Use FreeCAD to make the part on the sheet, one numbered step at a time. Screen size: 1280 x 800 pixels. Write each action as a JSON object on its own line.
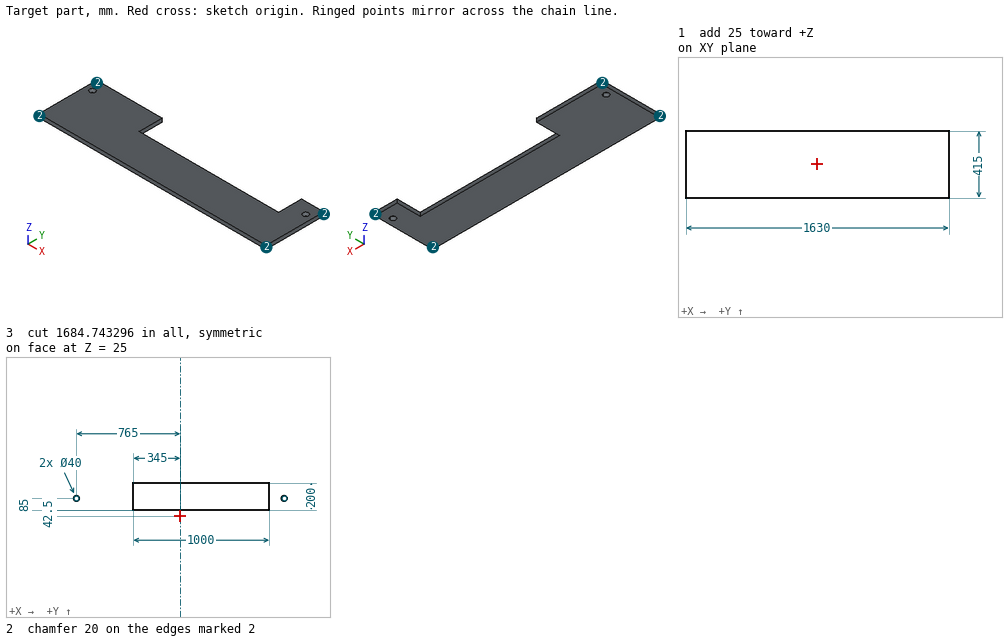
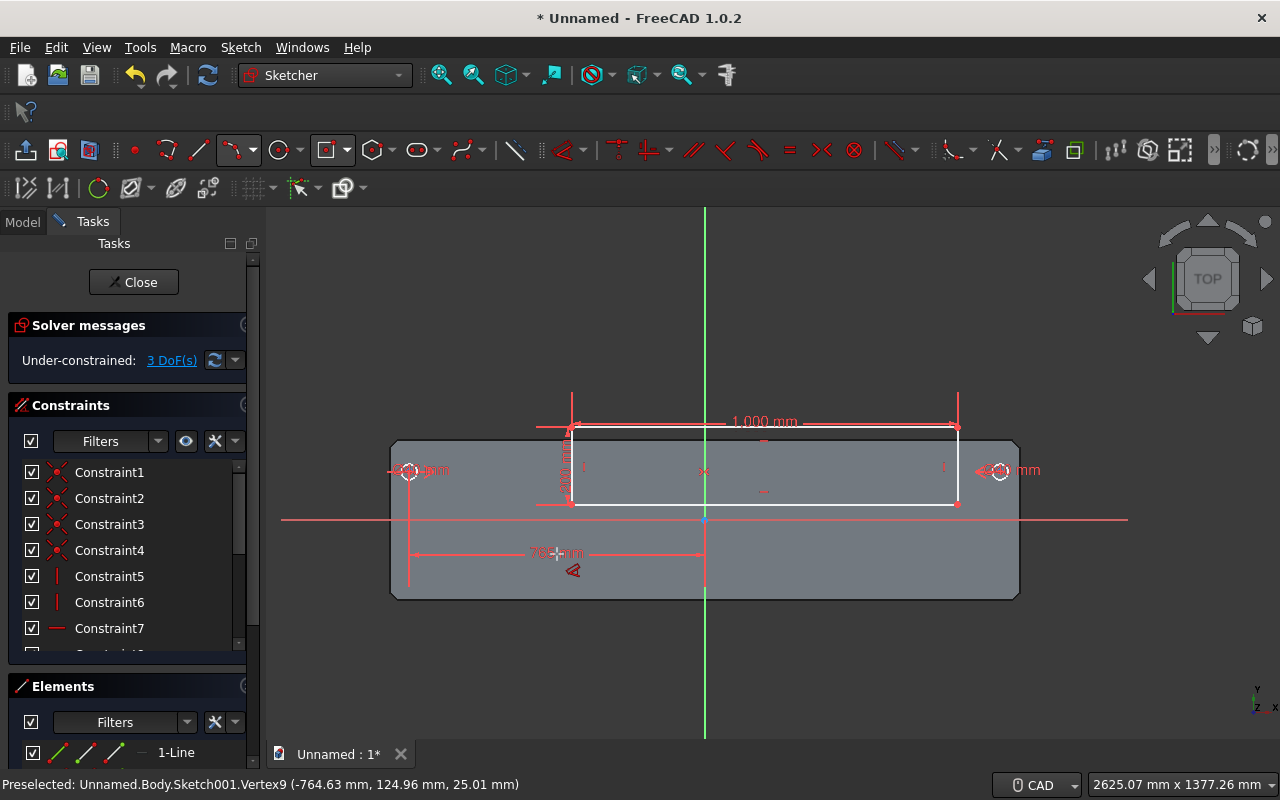
{"action": "left_click", "coordinate": [572, 505]}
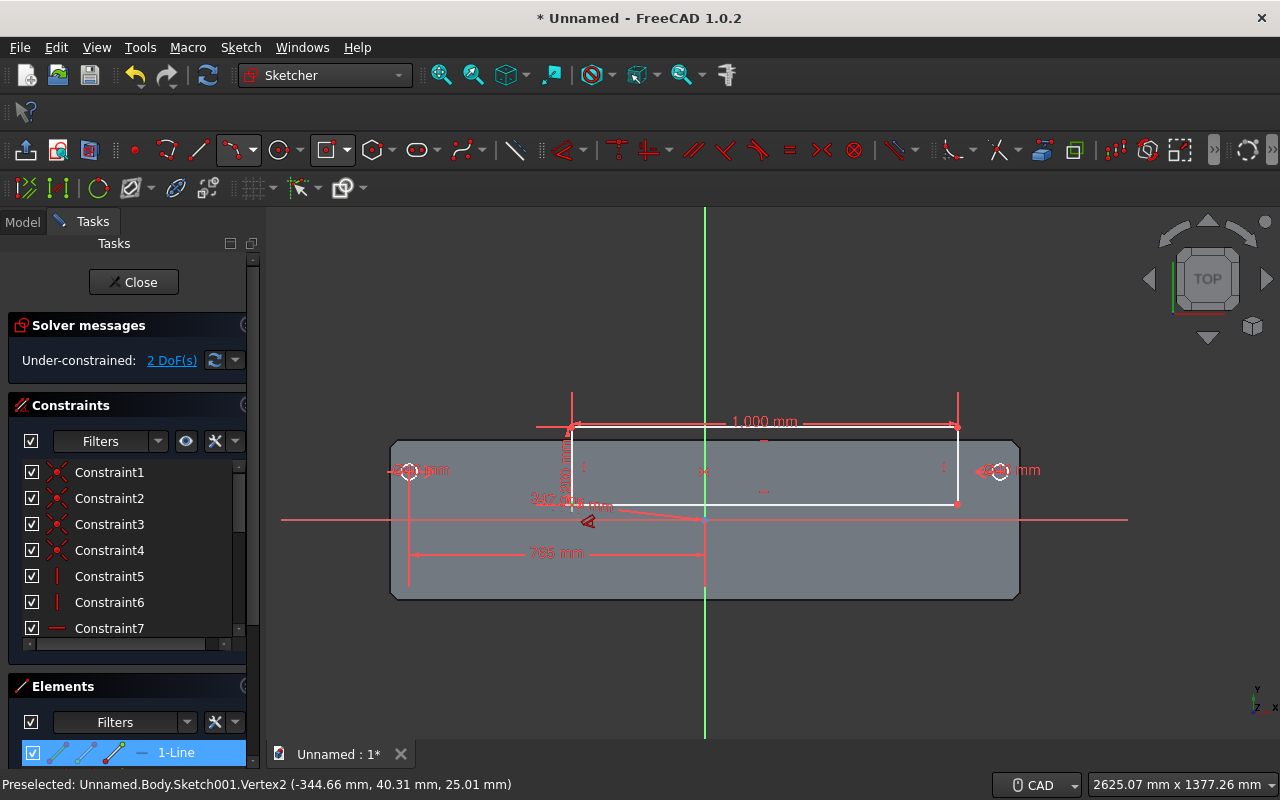
{"action": "left_click", "coordinate": [409, 472]}
{"action": "left_click", "coordinate": [375, 488]}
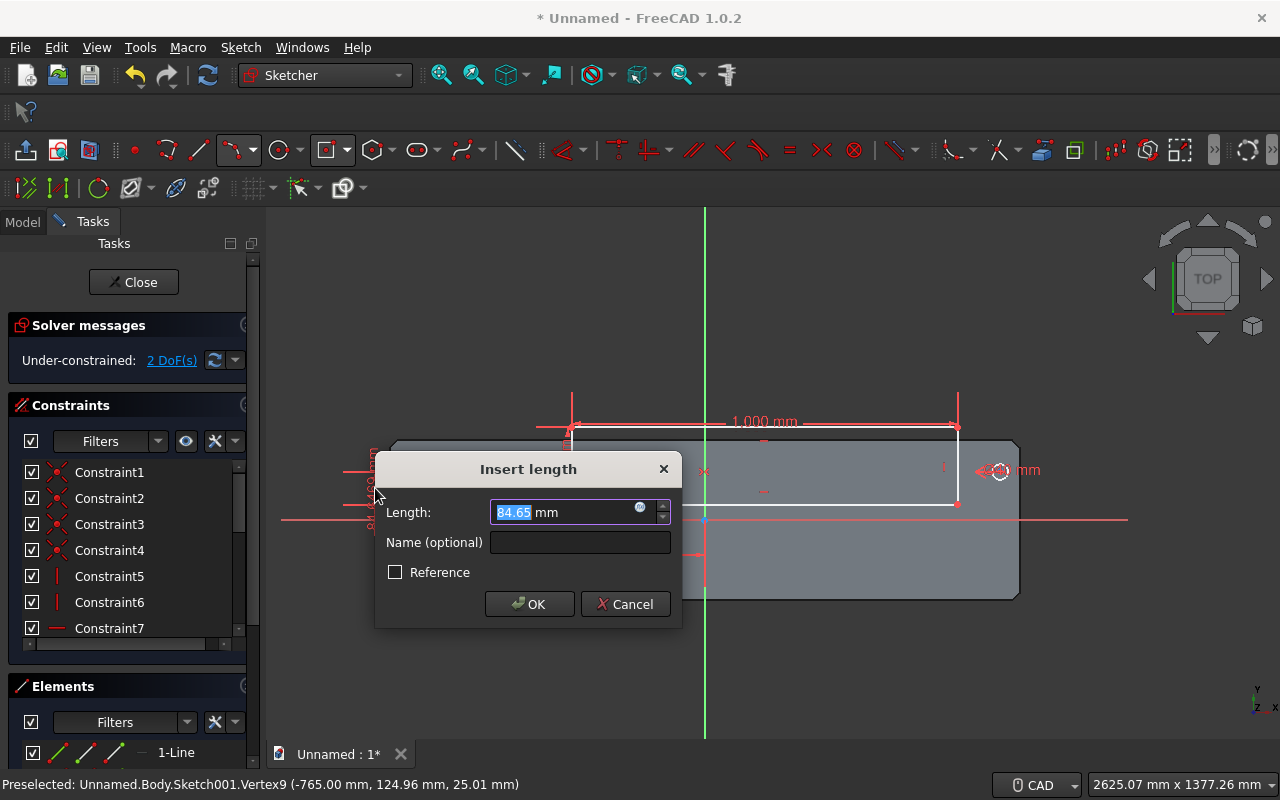
{"action": "type", "text": "85"}
{"action": "key", "text": "Return"}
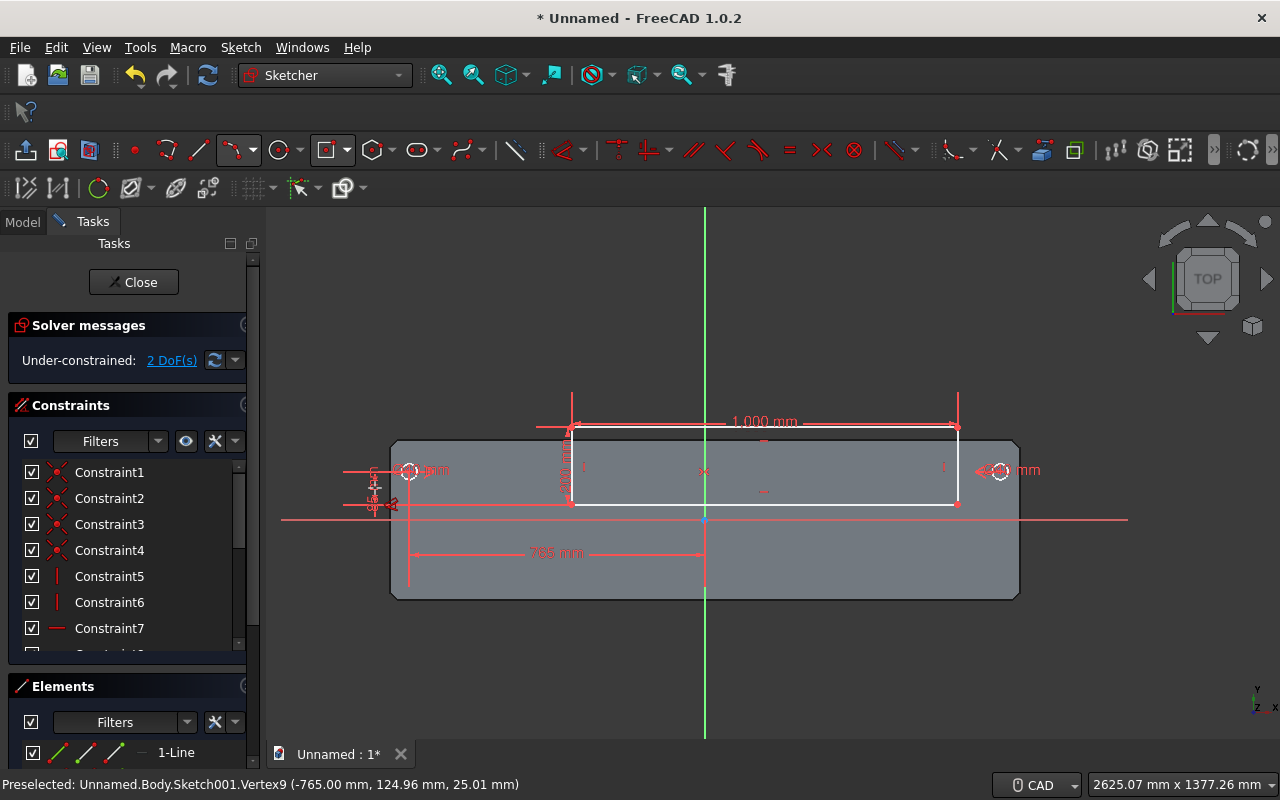
{"action": "left_click", "coordinate": [572, 427]}
{"action": "left_click", "coordinate": [638, 554]}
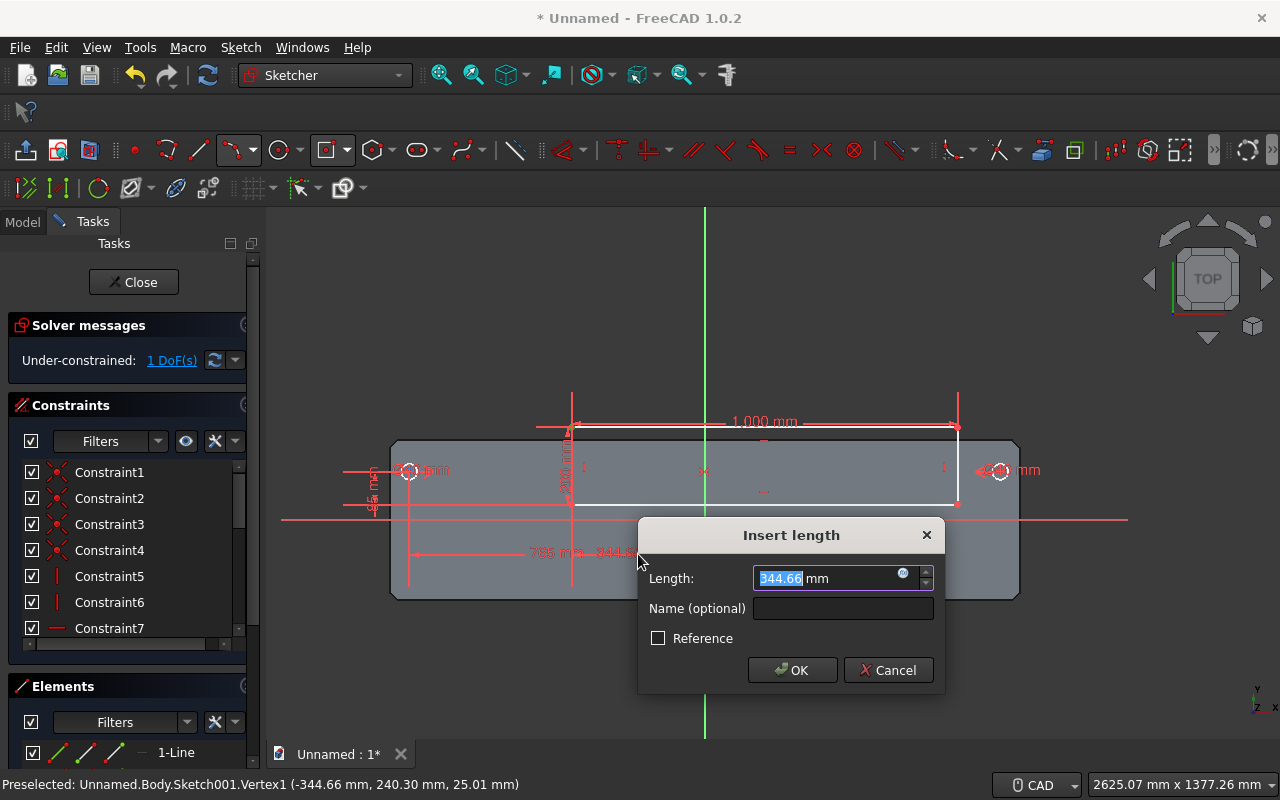
{"action": "type", "text": "345"}
{"action": "key", "text": "Return"}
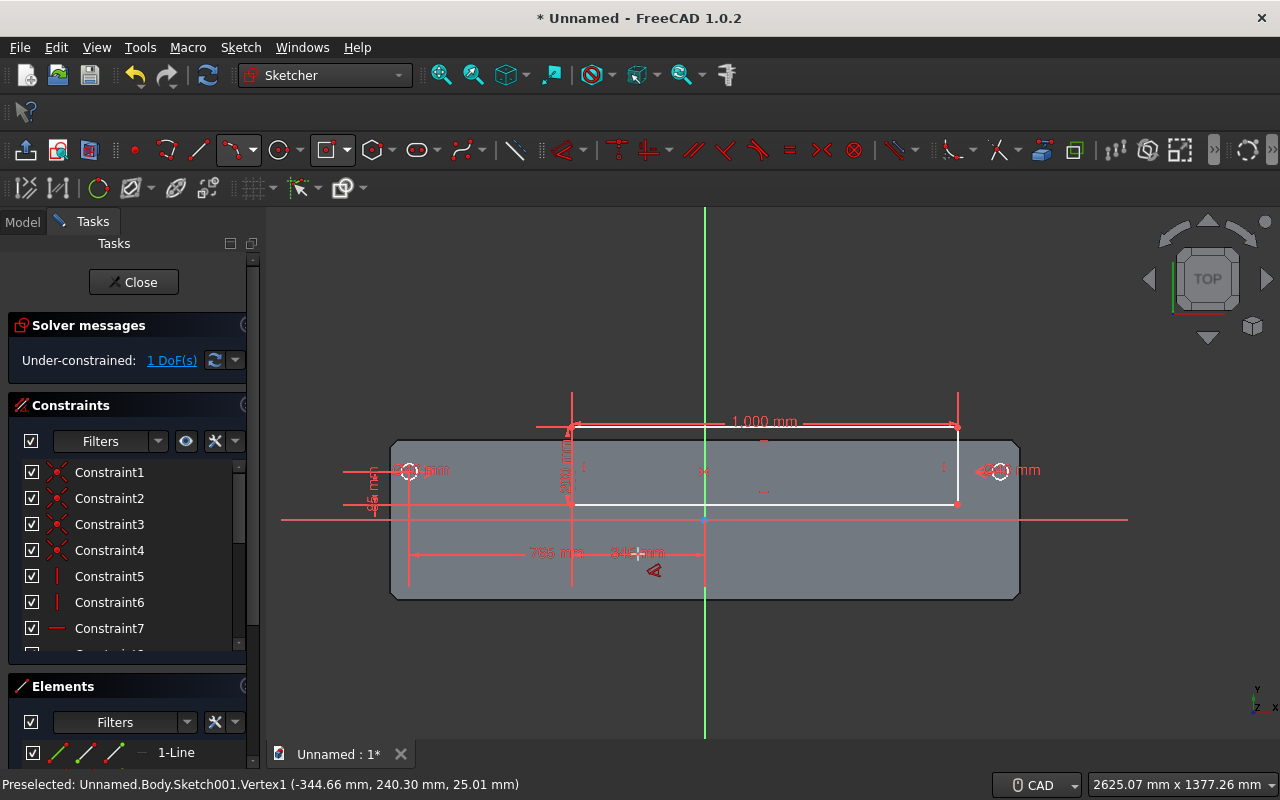
{"action": "scroll", "coordinate": [572, 505], "scroll_direction": "up", "scroll_amount": 5}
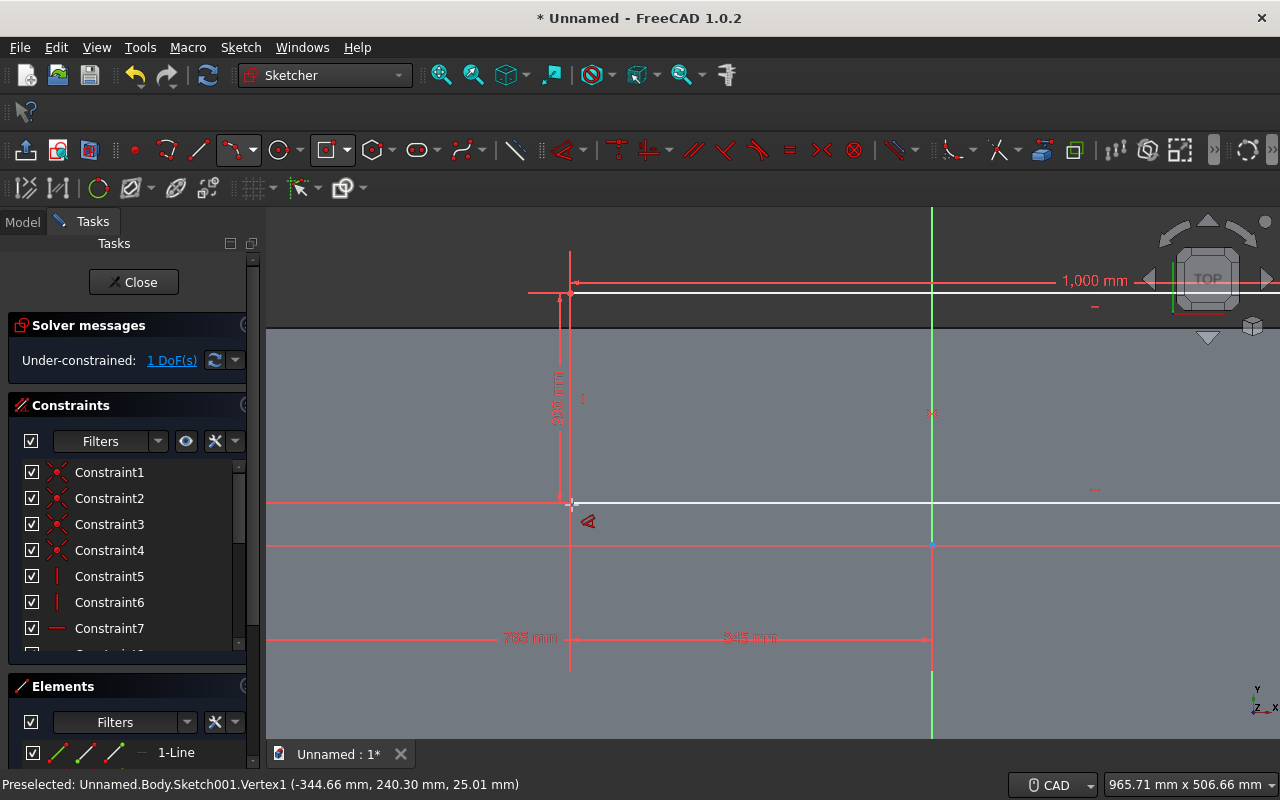
{"action": "left_click", "coordinate": [570, 503]}
{"action": "left_click", "coordinate": [536, 524]}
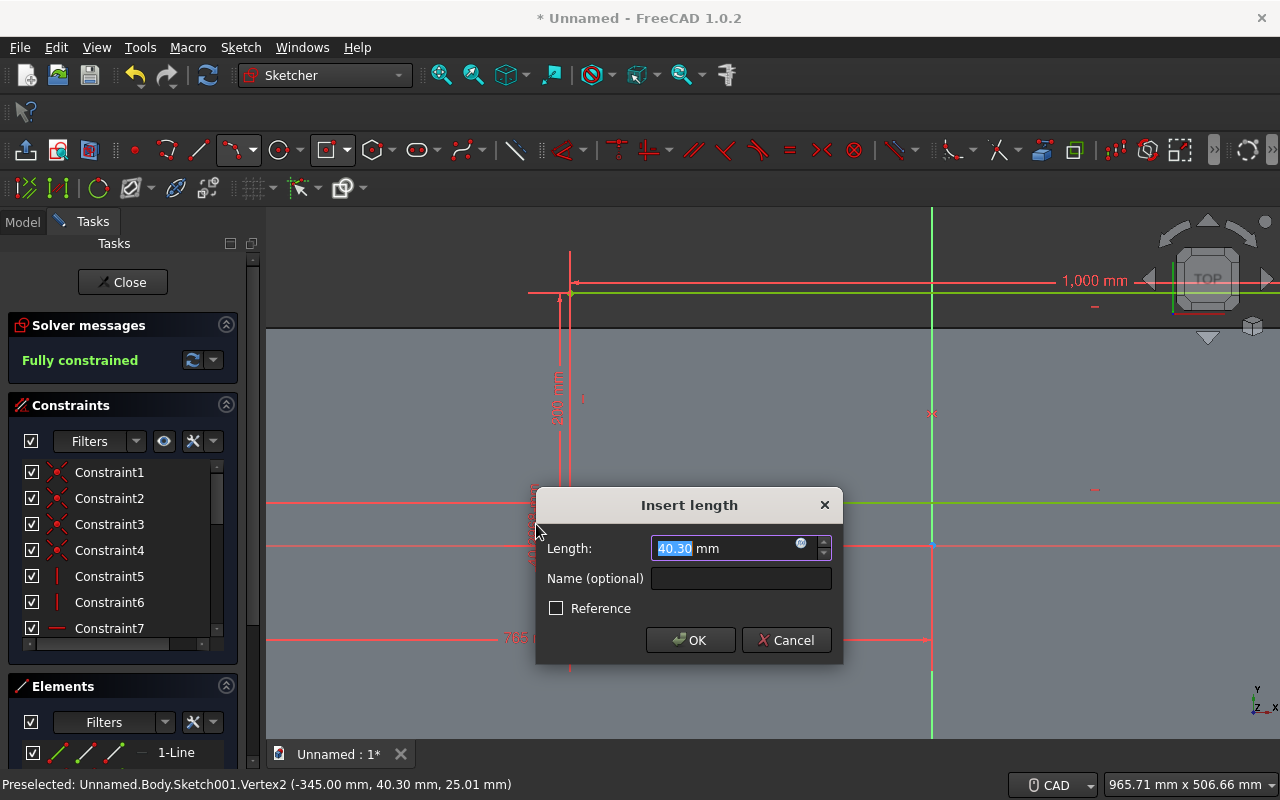
{"action": "type", "text": "42.5"}
{"action": "key", "text": "Return"}
{"action": "key", "text": "Escape"}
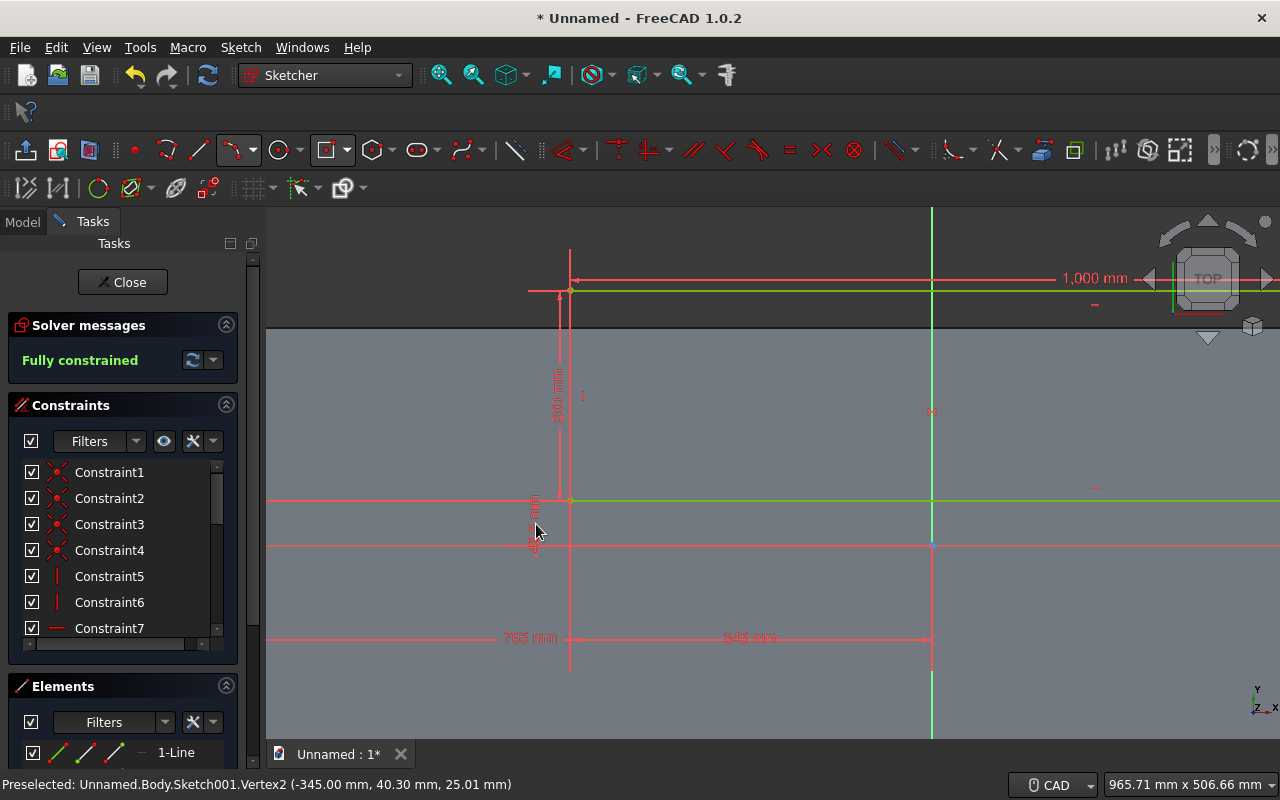
{"action": "left_click", "coordinate": [123, 282]}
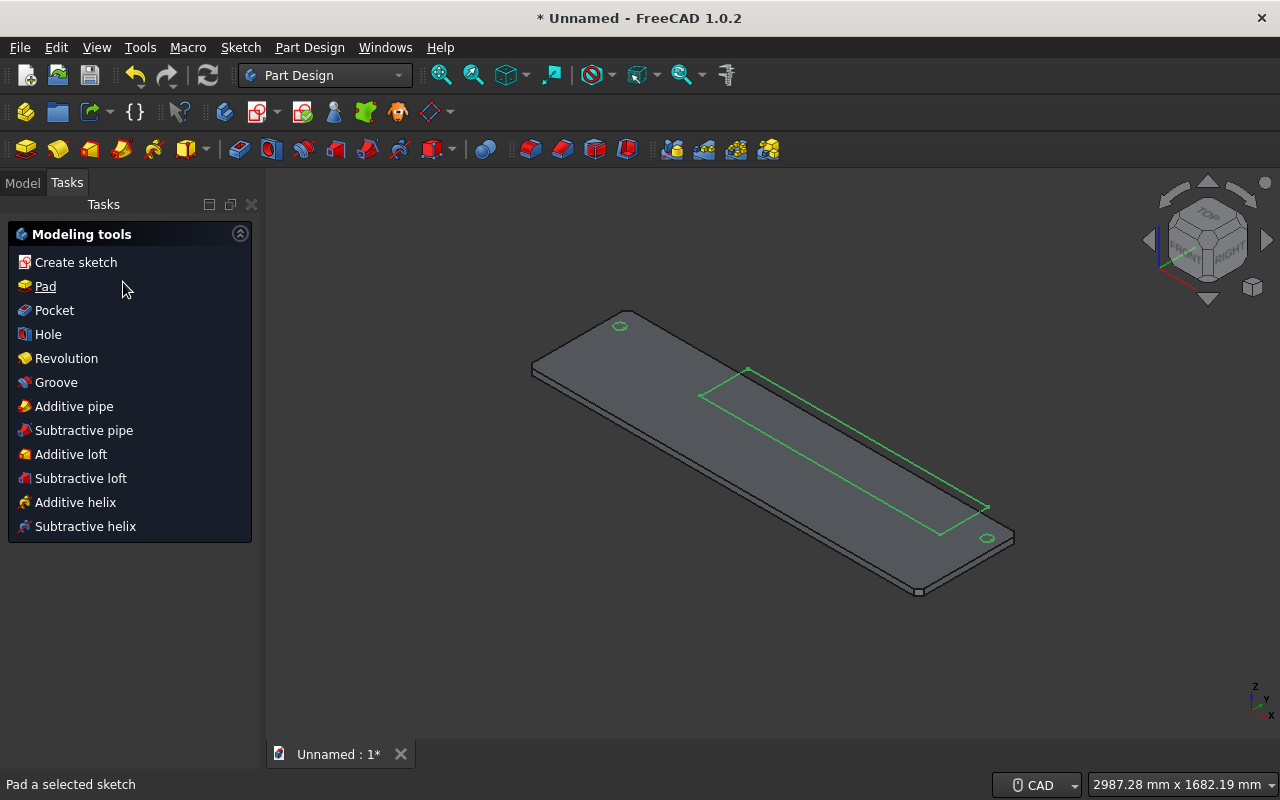
{"action": "left_click", "coordinate": [240, 150]}